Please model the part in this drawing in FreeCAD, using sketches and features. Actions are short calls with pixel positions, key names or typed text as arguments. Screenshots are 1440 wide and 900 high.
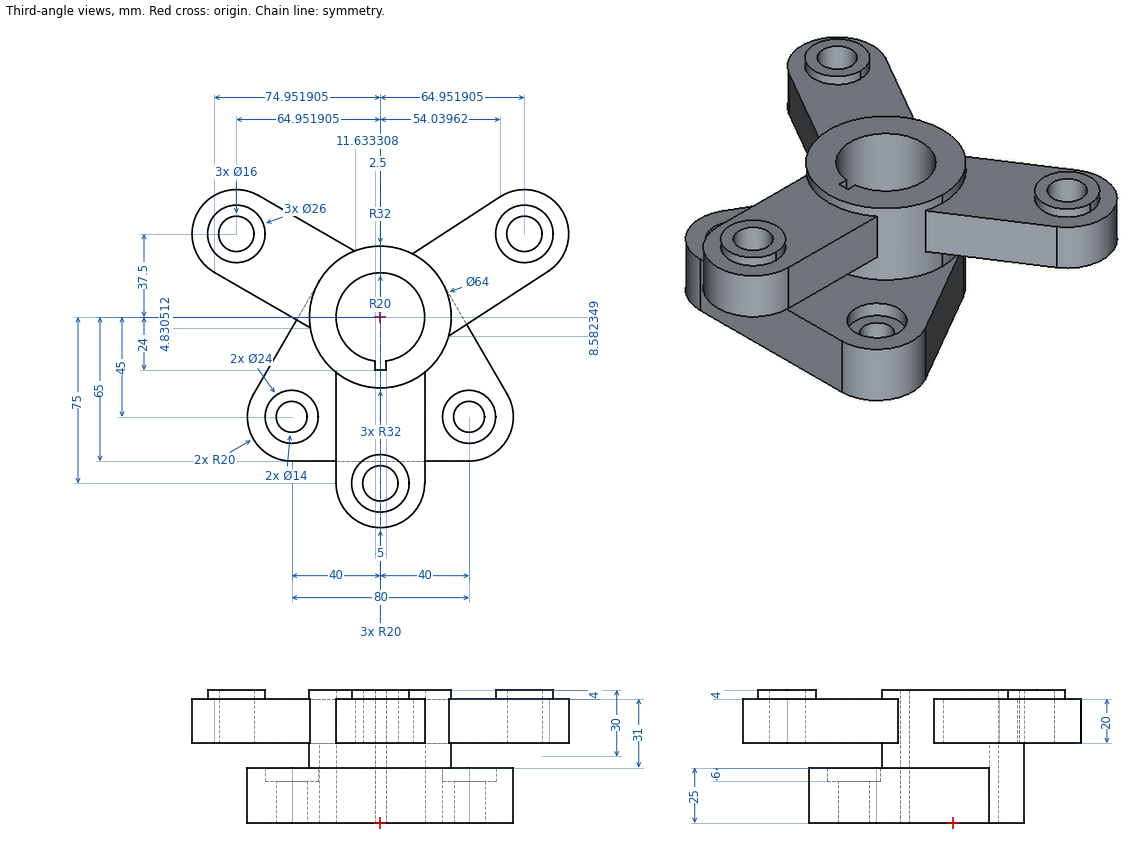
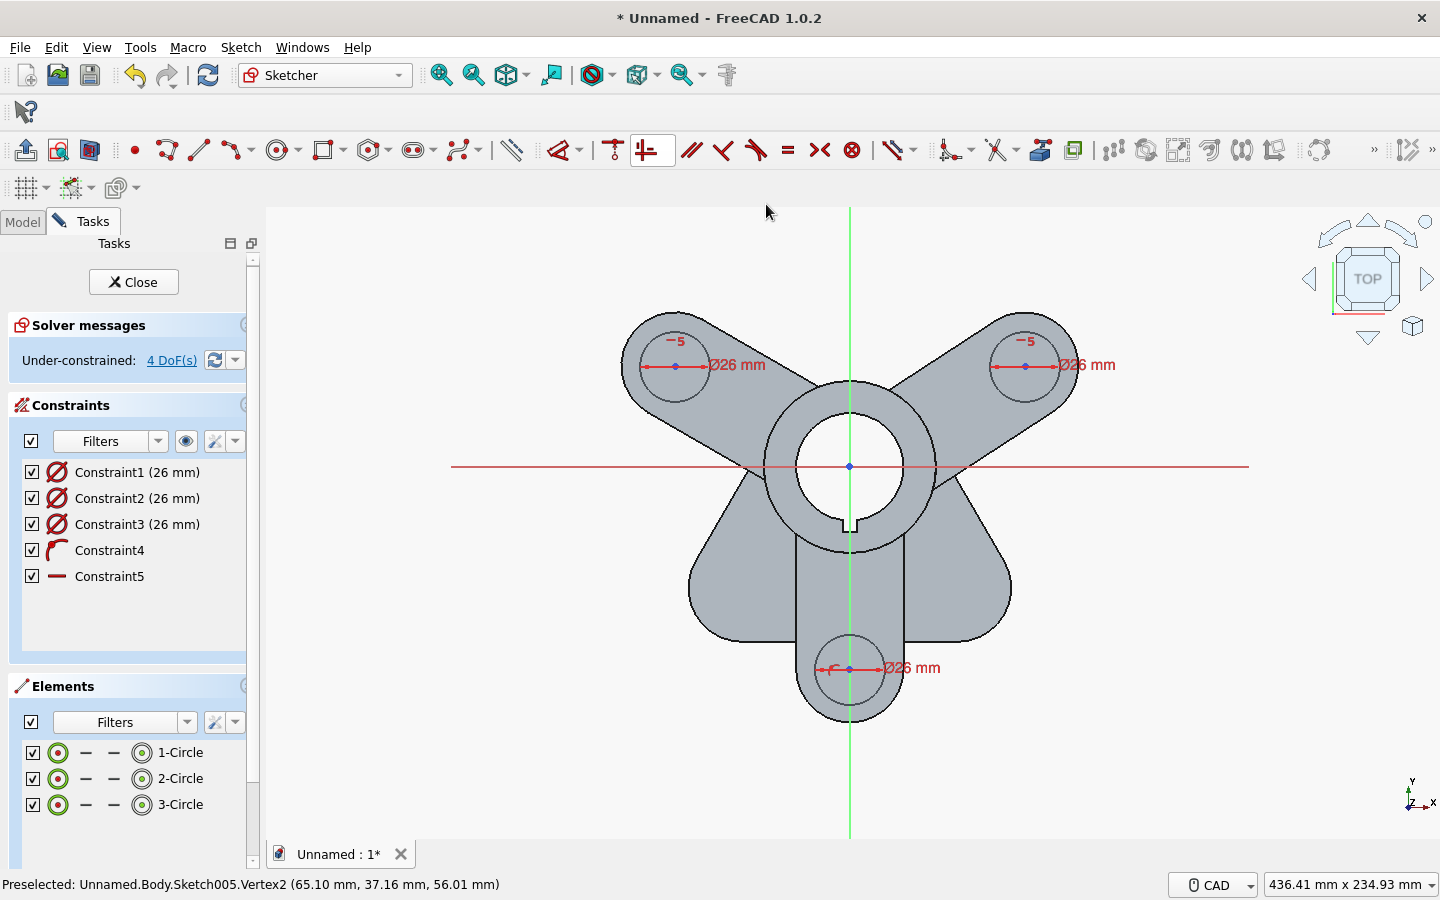
click(558, 150)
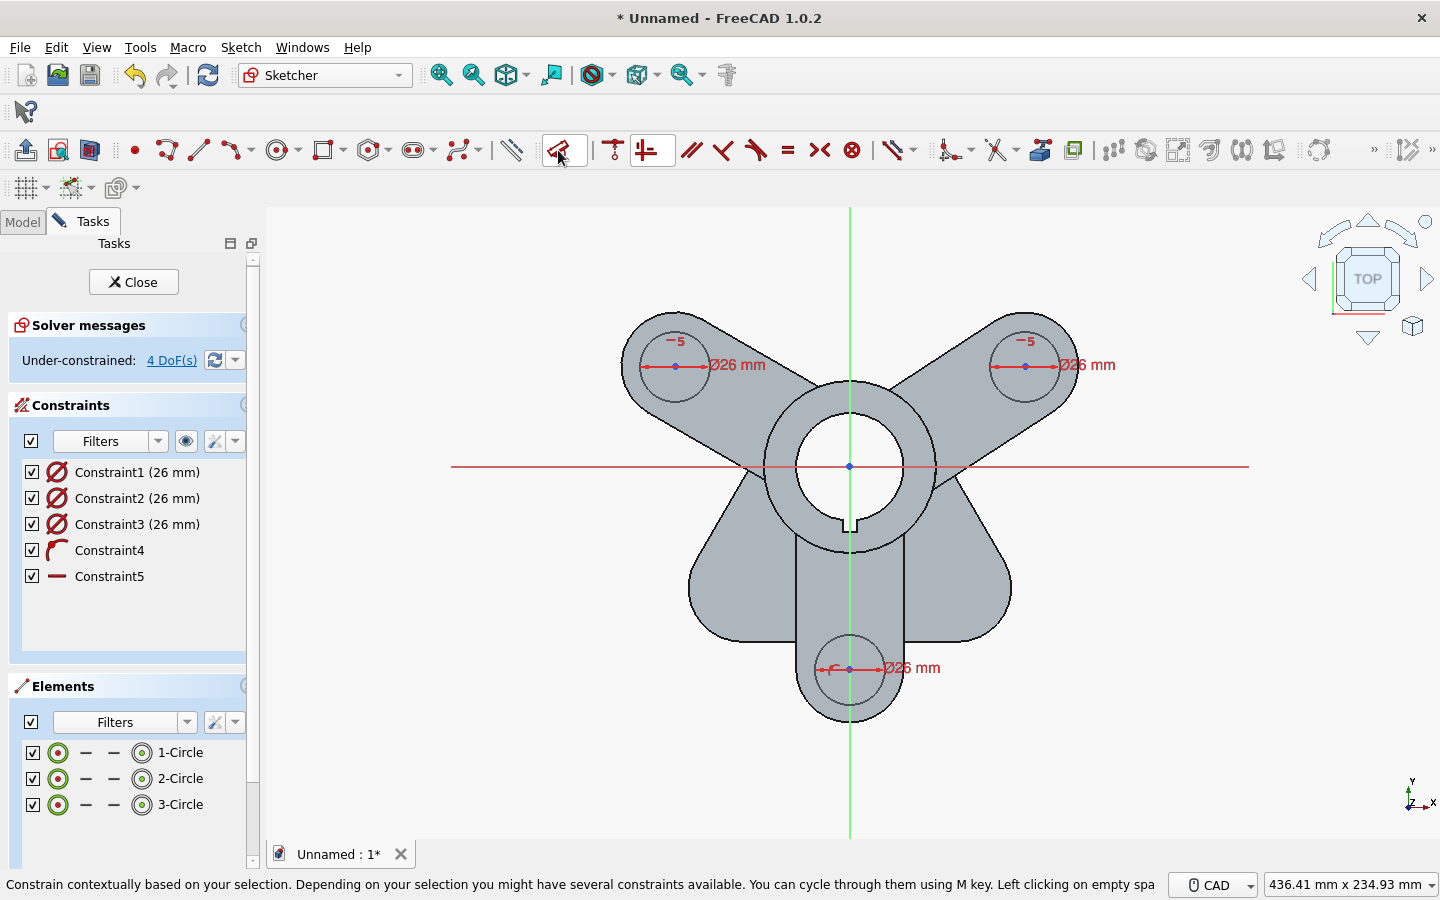
click(850, 670)
click(884, 568)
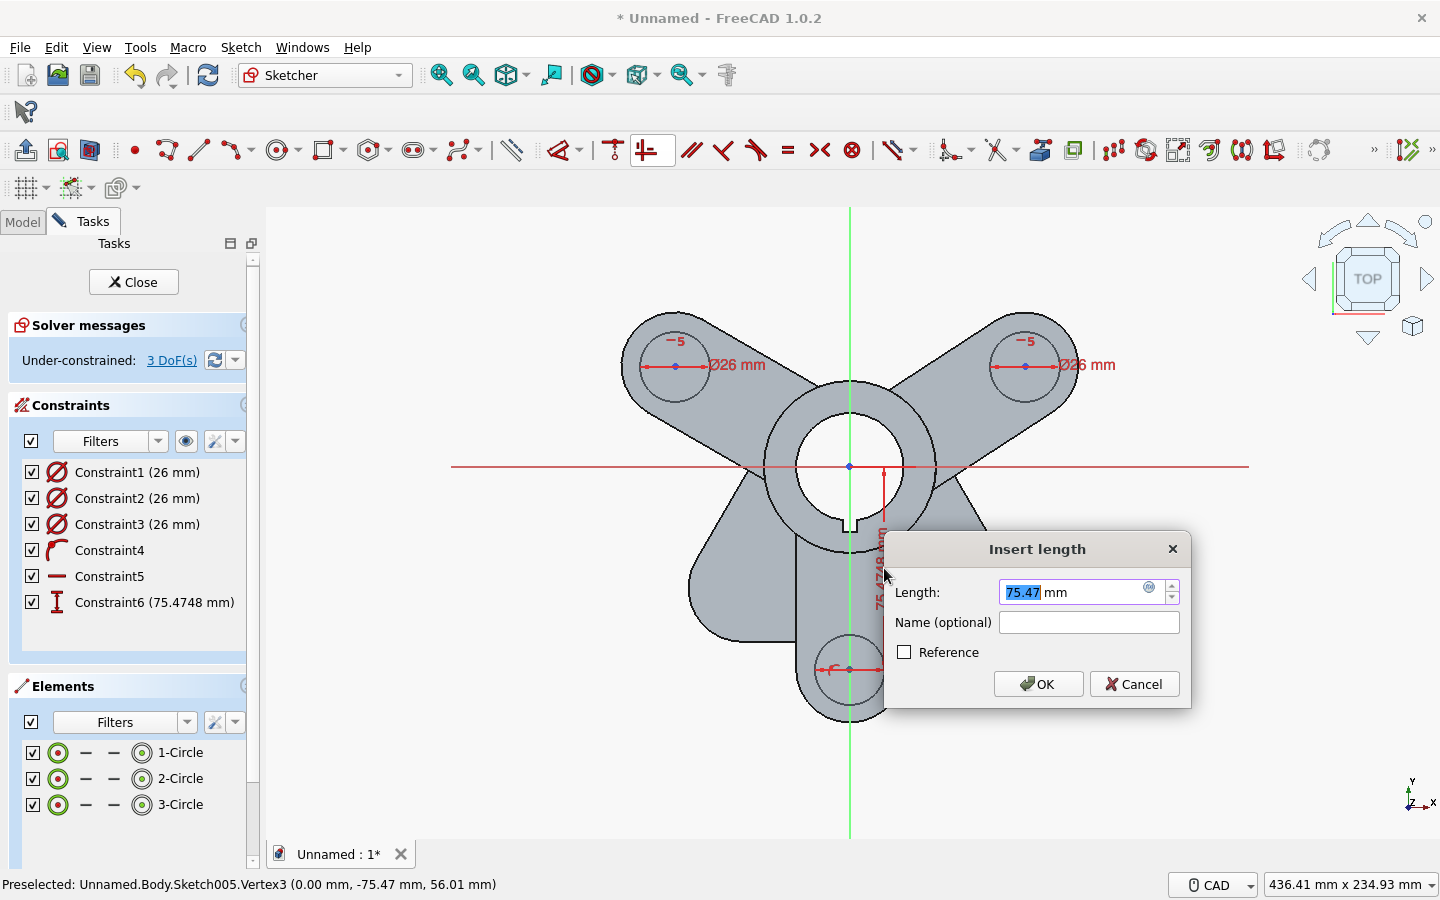
text(75)
key(Return)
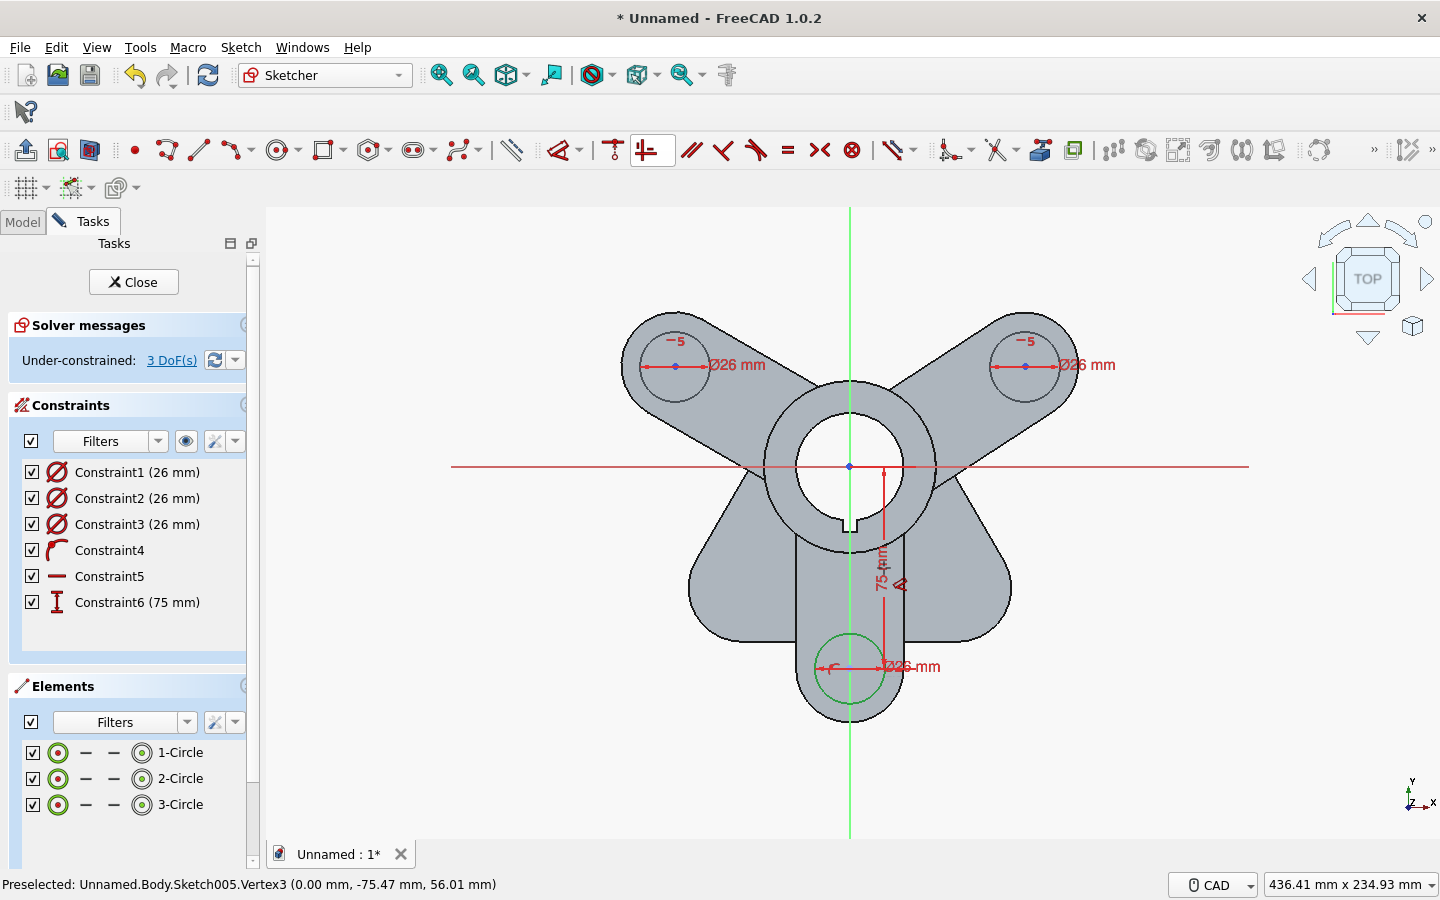
click(675, 367)
click(641, 417)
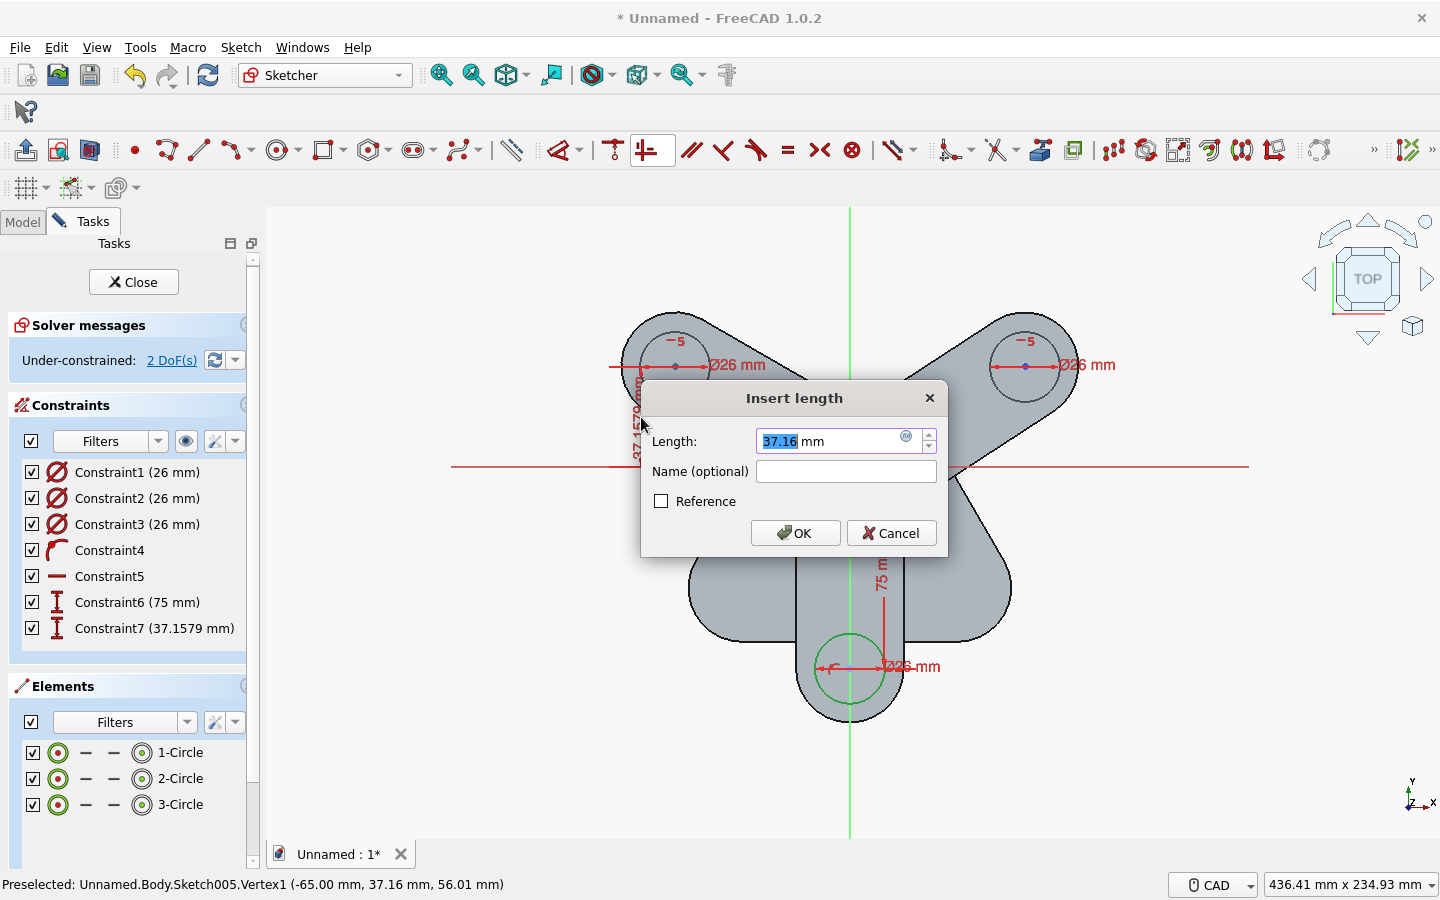
text(37.5)
key(Return)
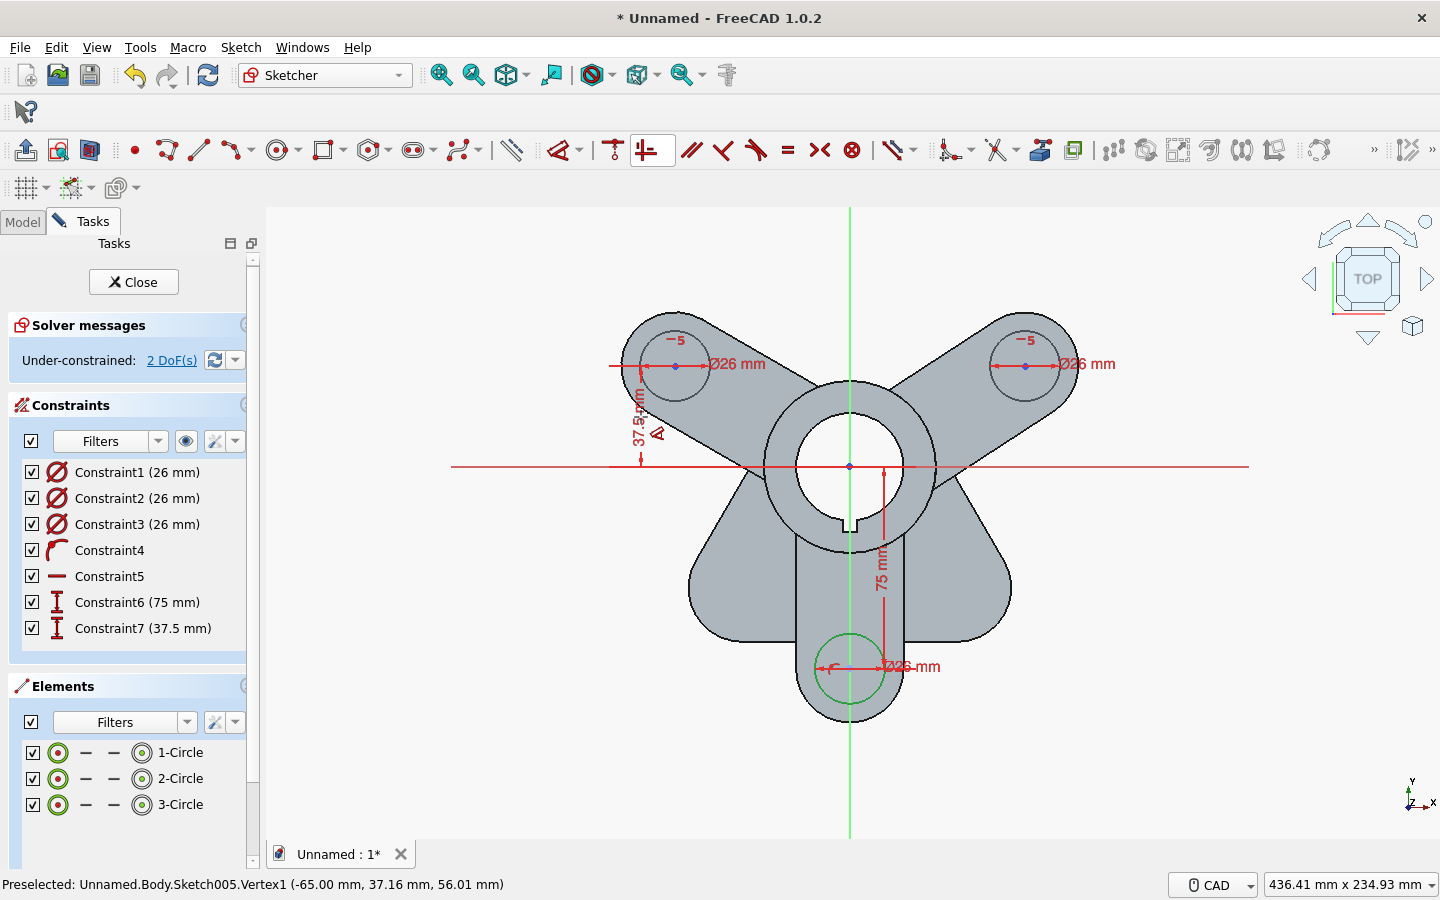
click(675, 366)
click(762, 332)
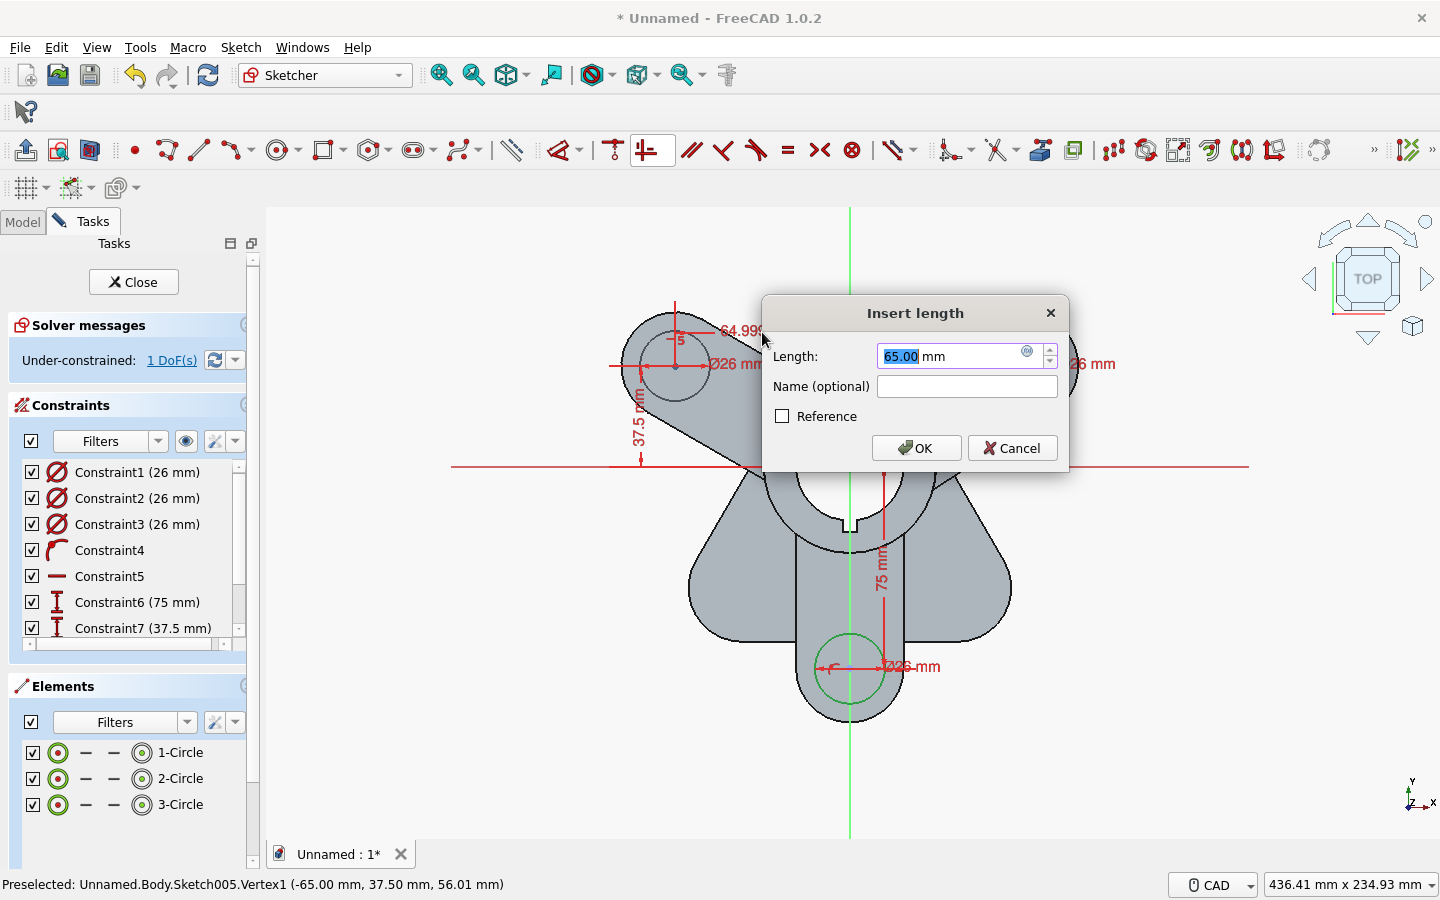
text(64.951905)
key(Return)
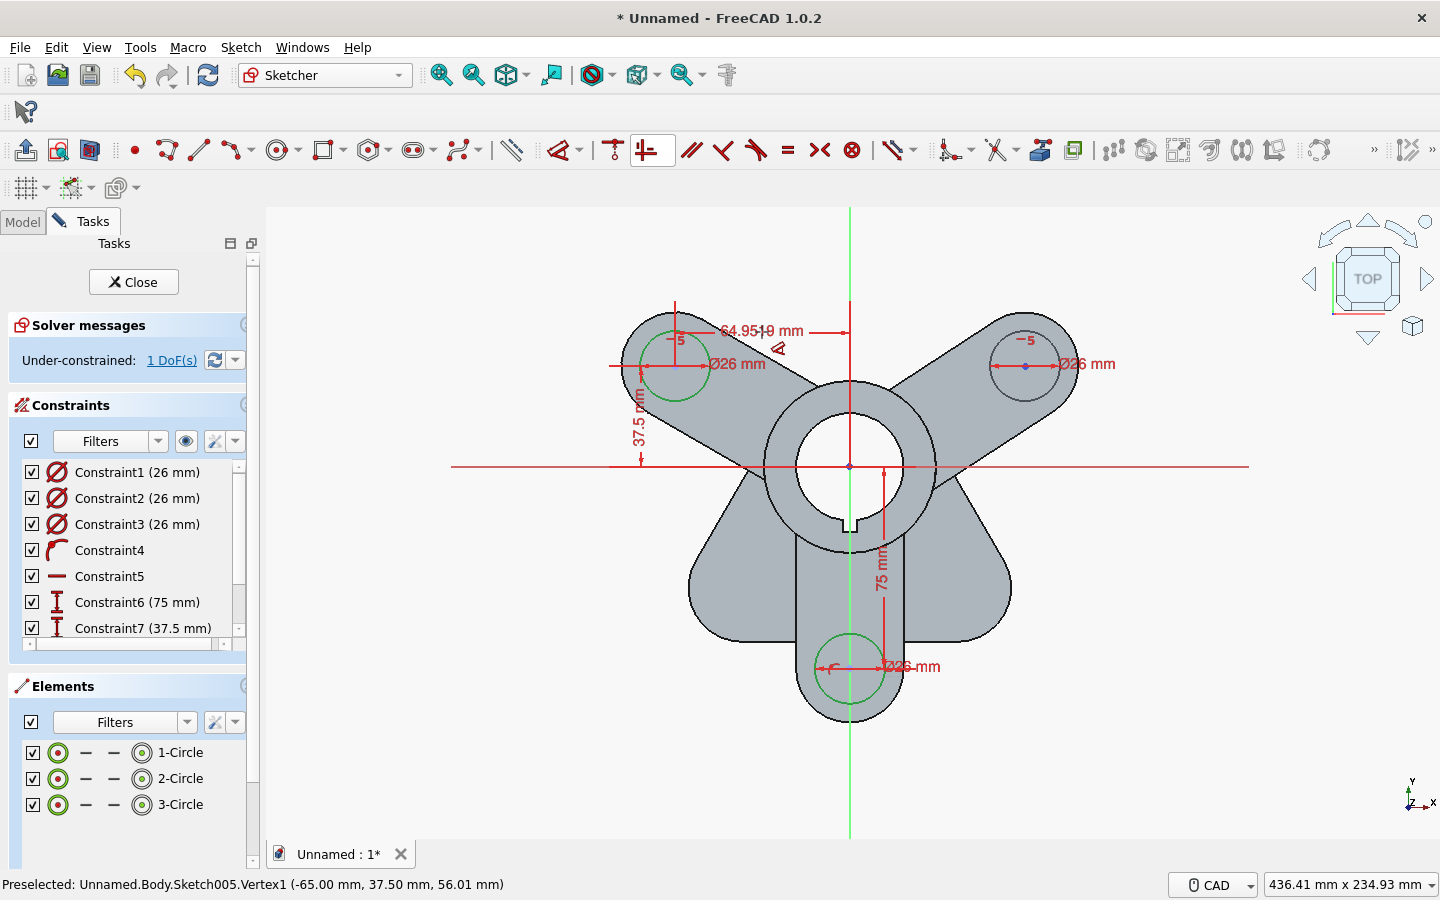
click(1025, 366)
click(937, 332)